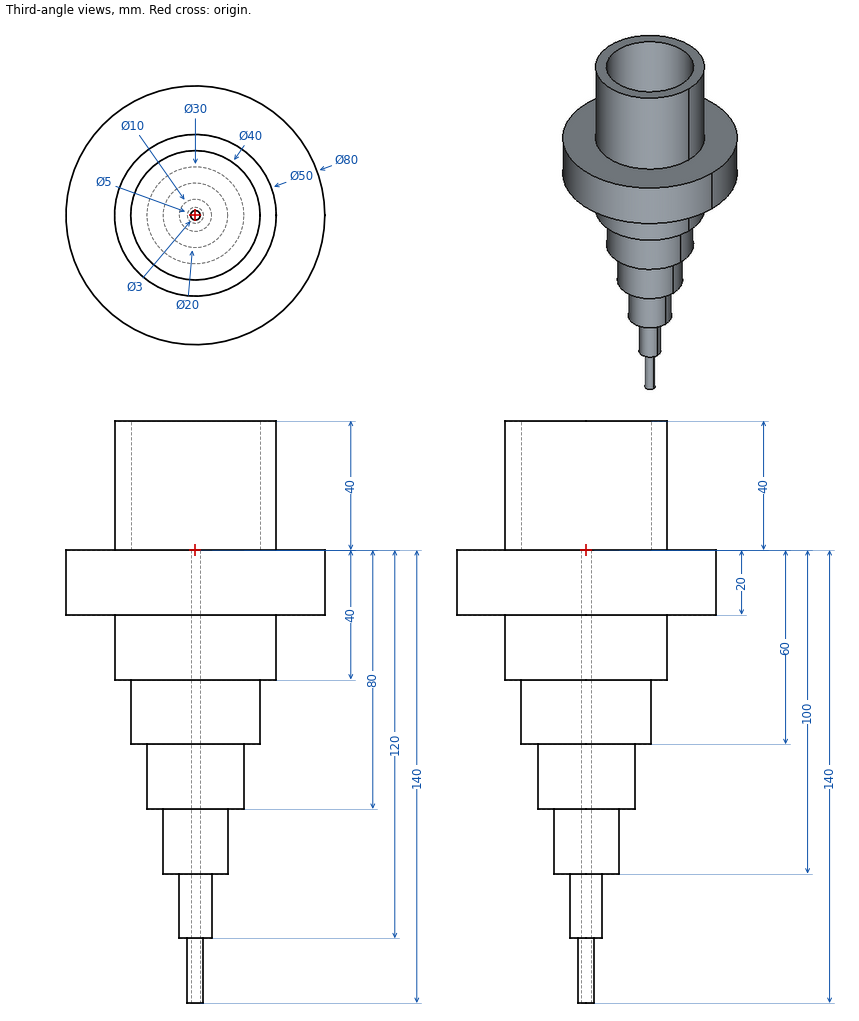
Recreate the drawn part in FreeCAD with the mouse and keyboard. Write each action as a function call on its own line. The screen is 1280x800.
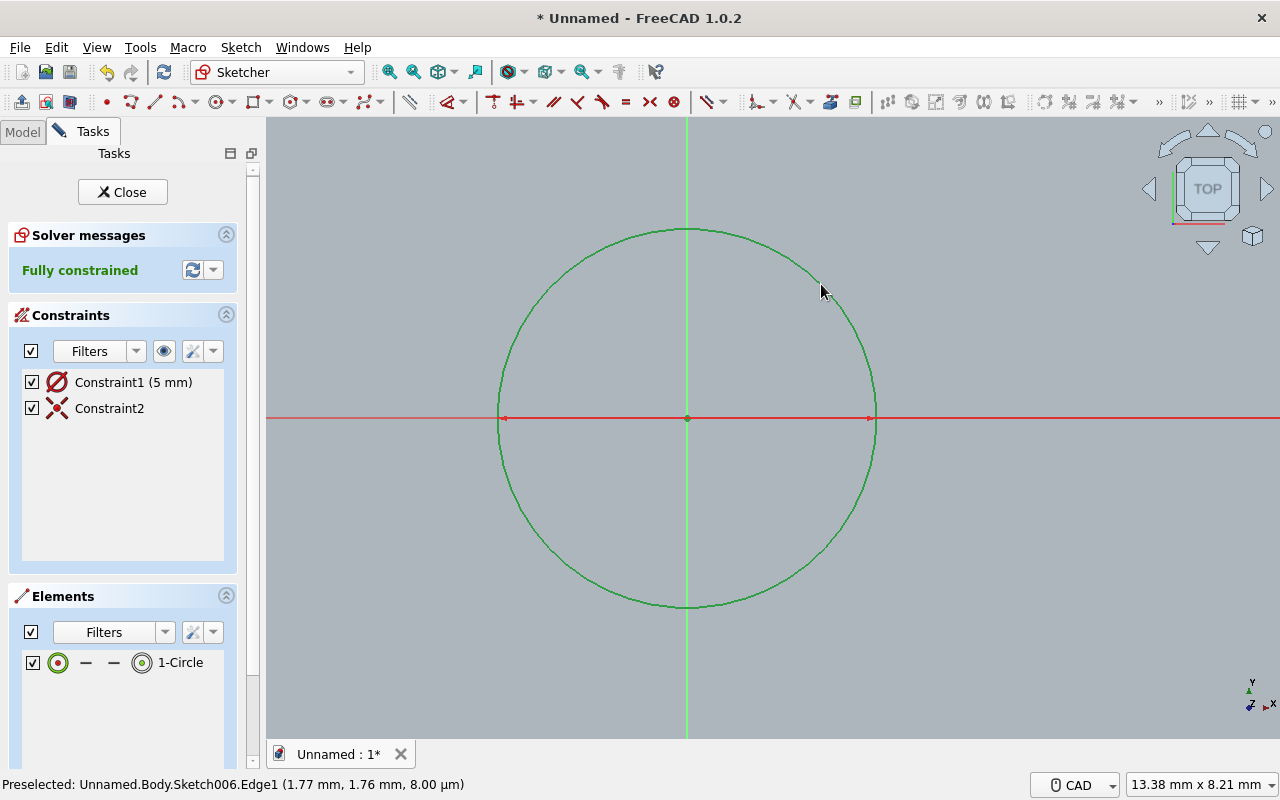
click(123, 192)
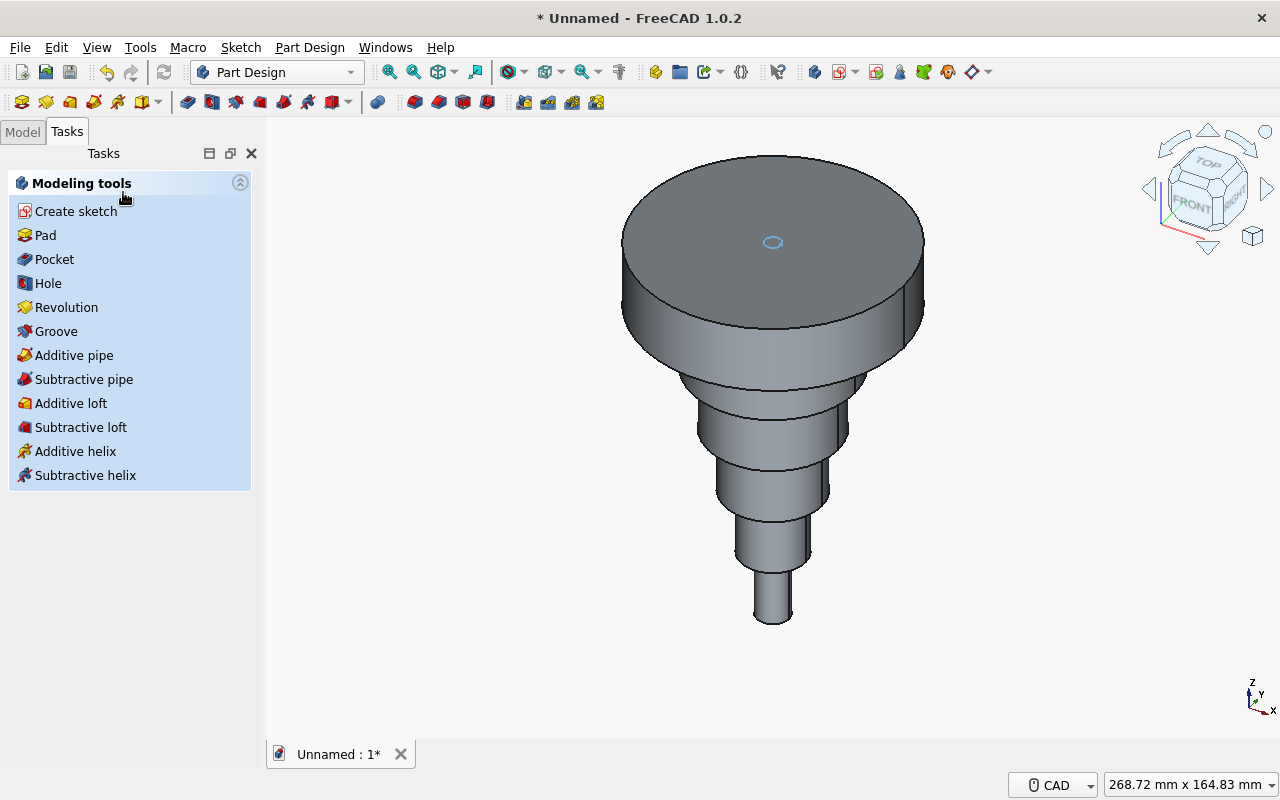
click(22, 102)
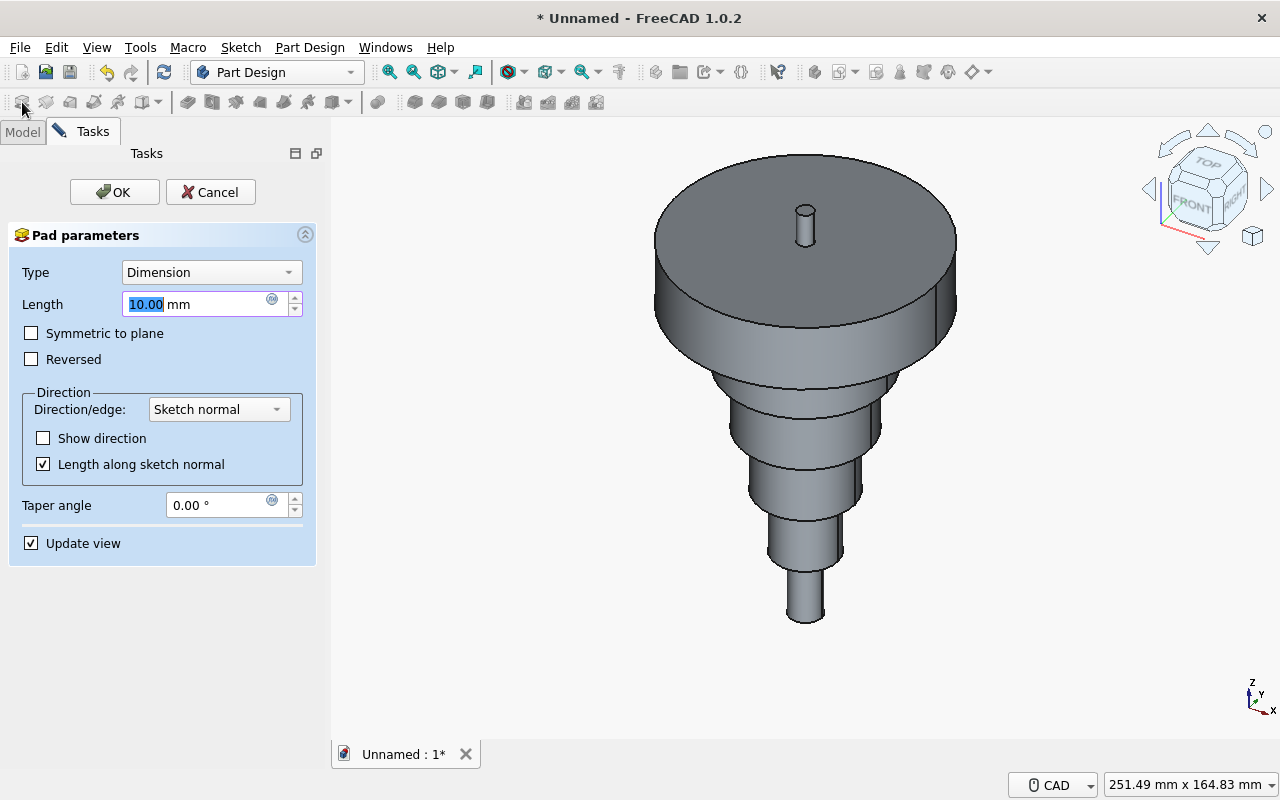
text(140)
key(Tab)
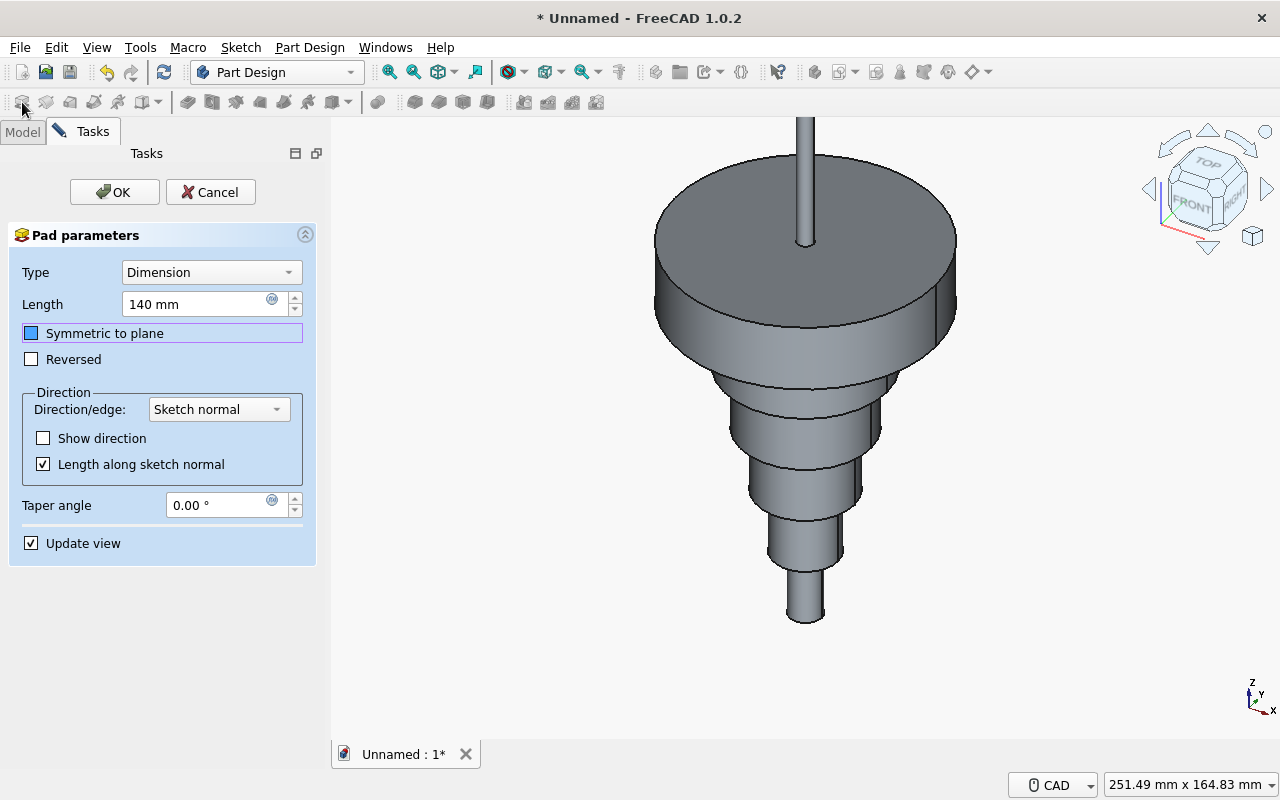
click(30, 359)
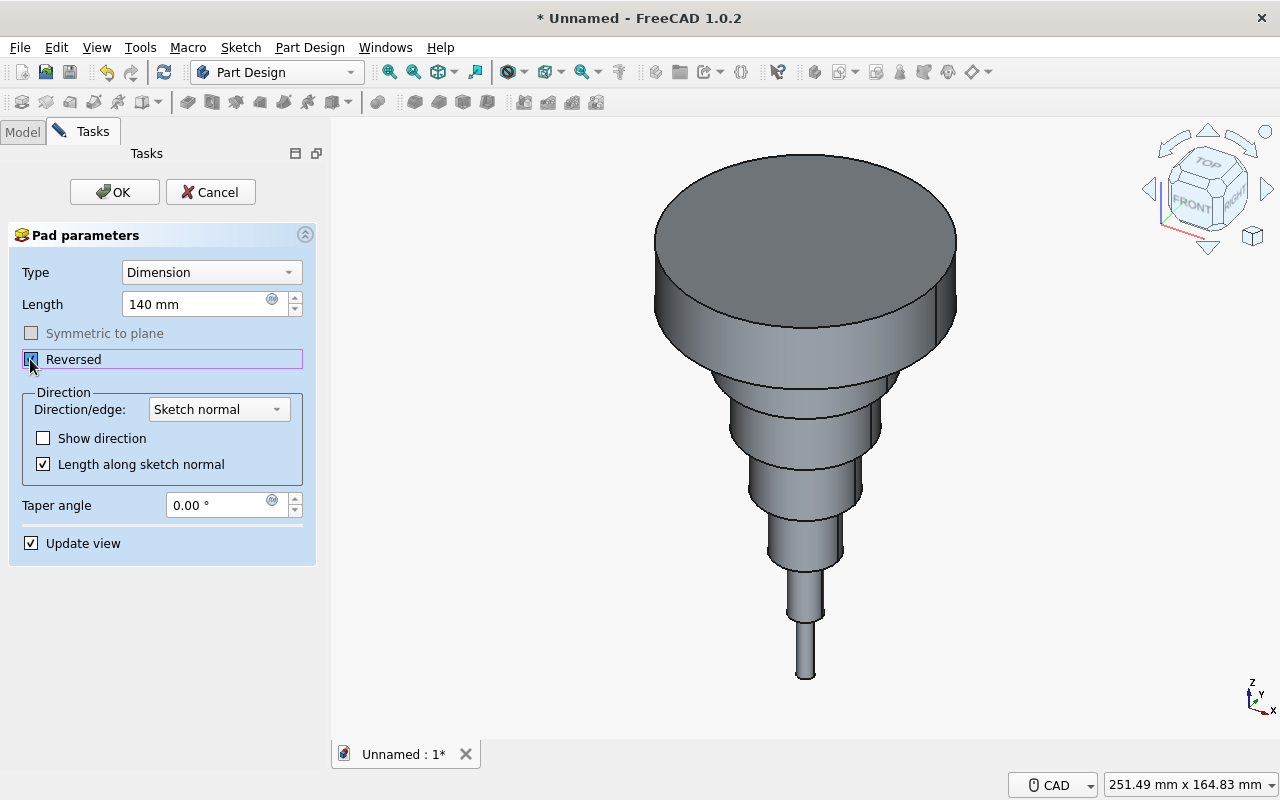
click(115, 192)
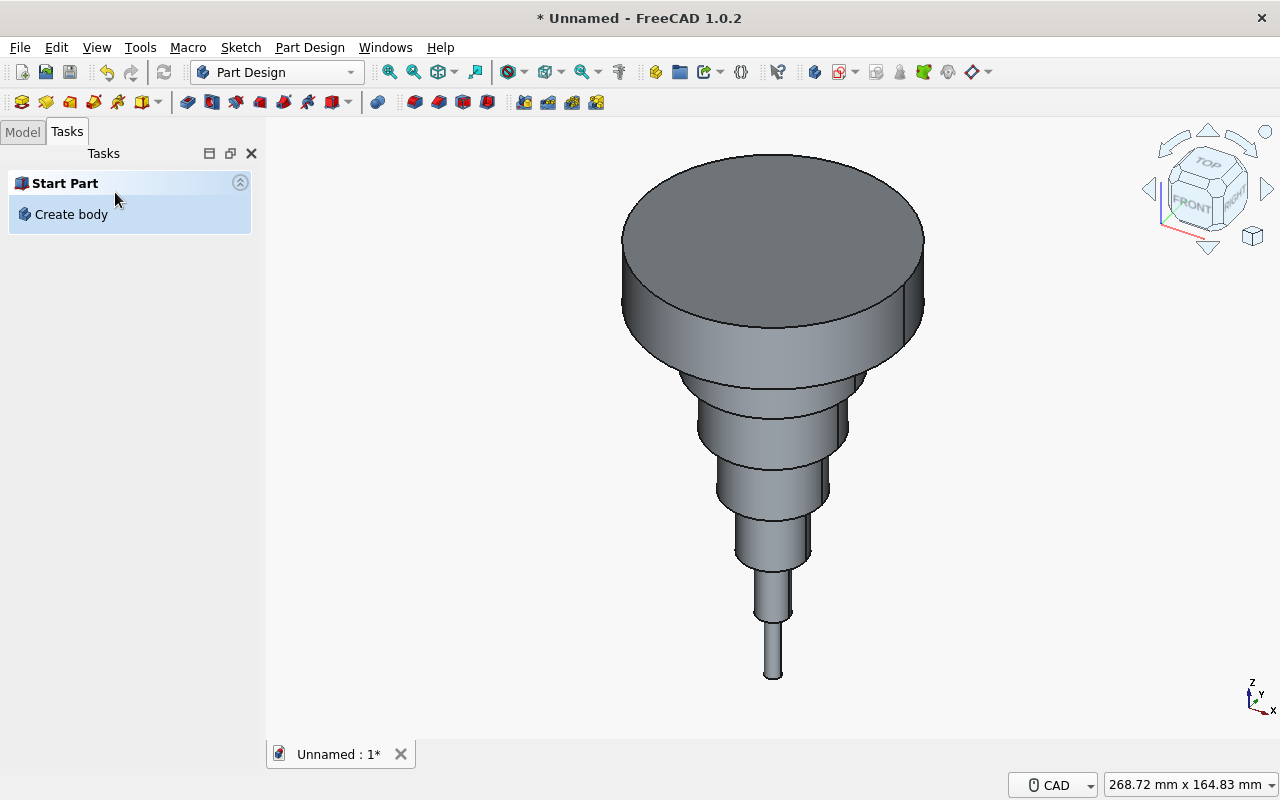
key(v)
key(f)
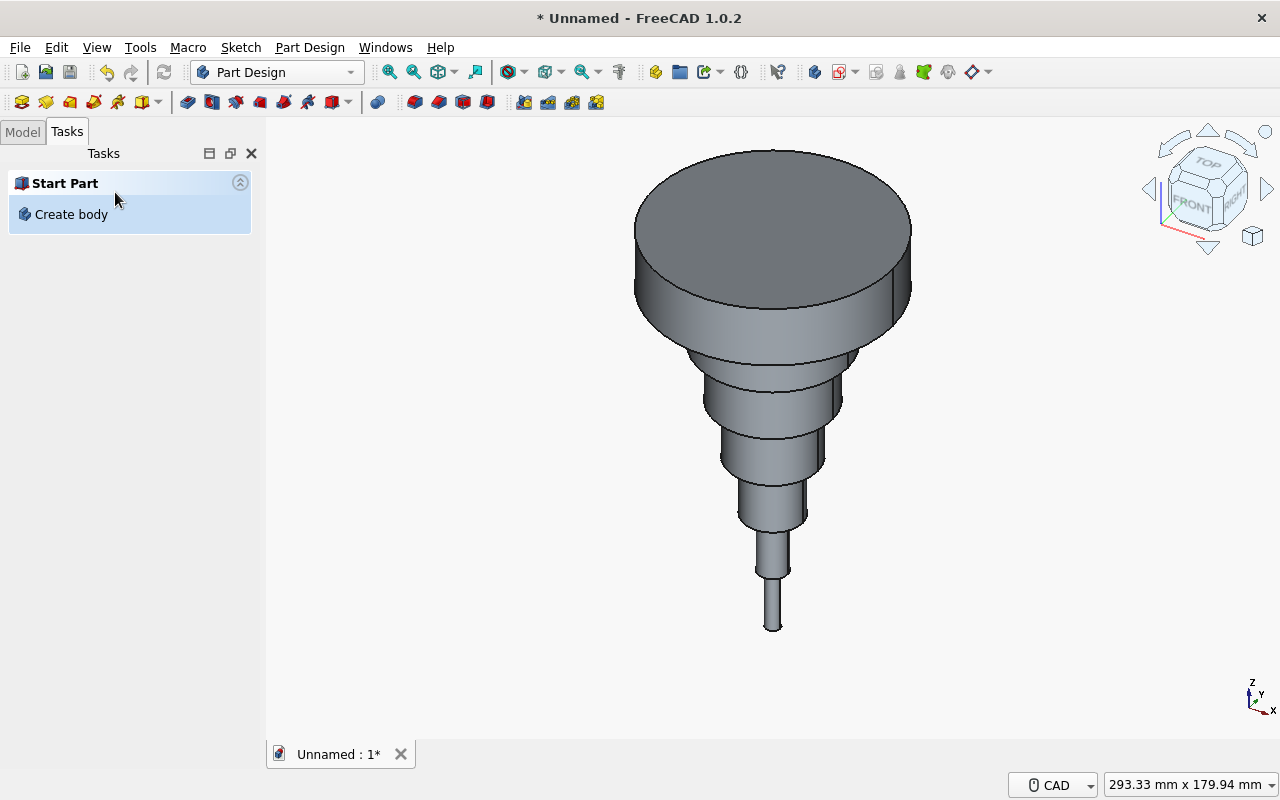
click(23, 131)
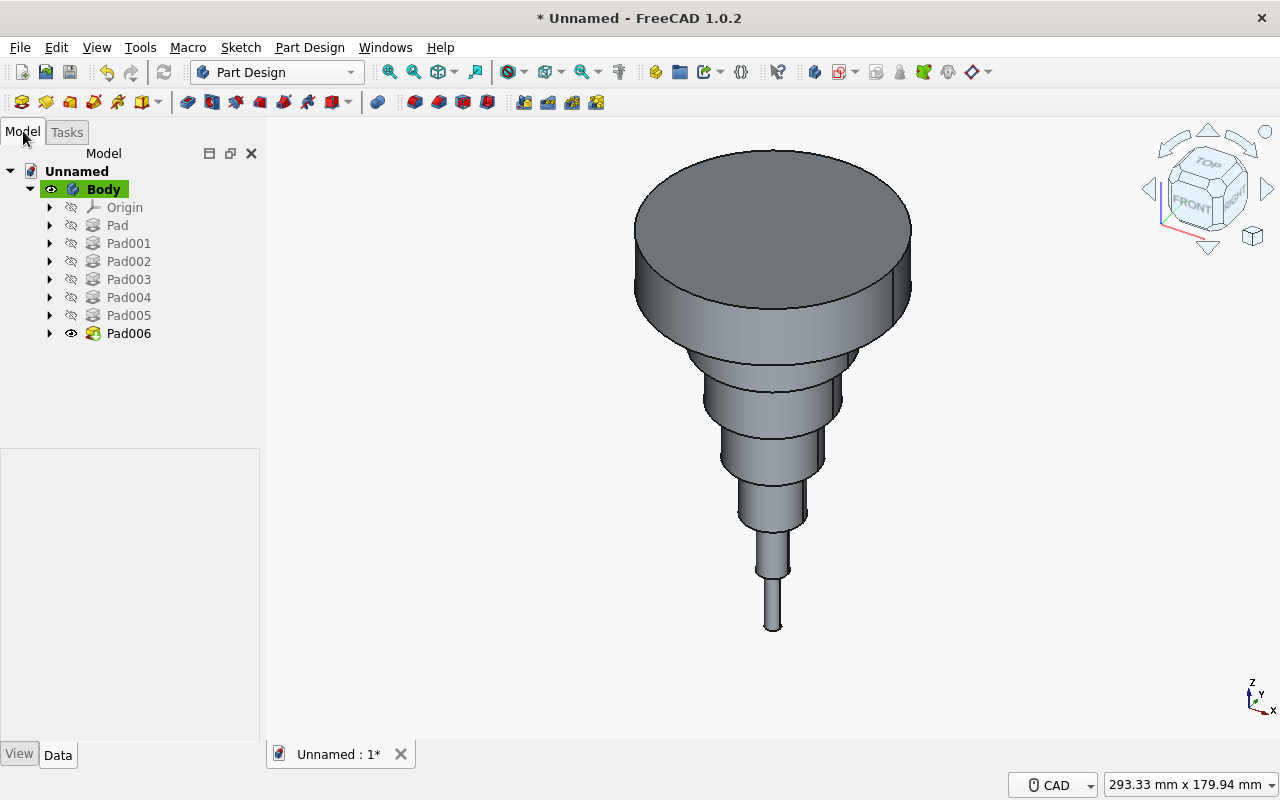
click(50, 207)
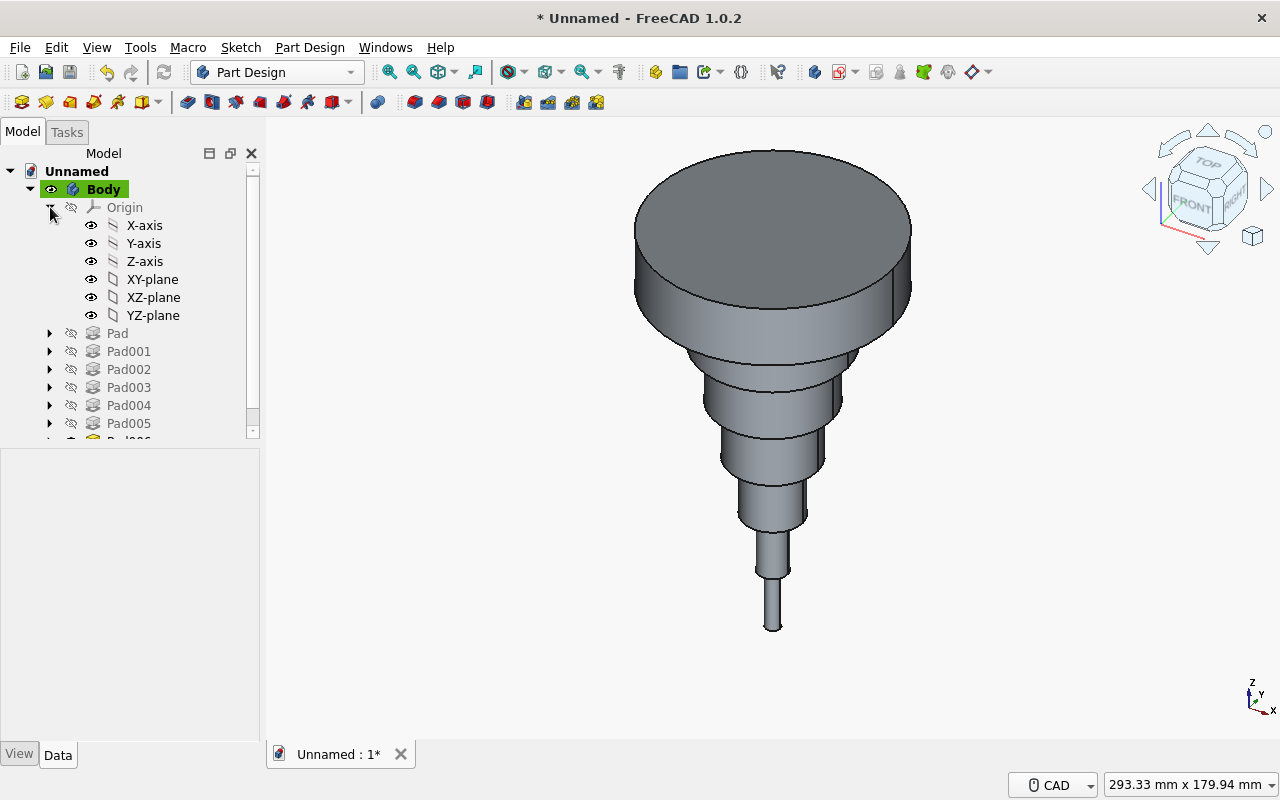
click(136, 279)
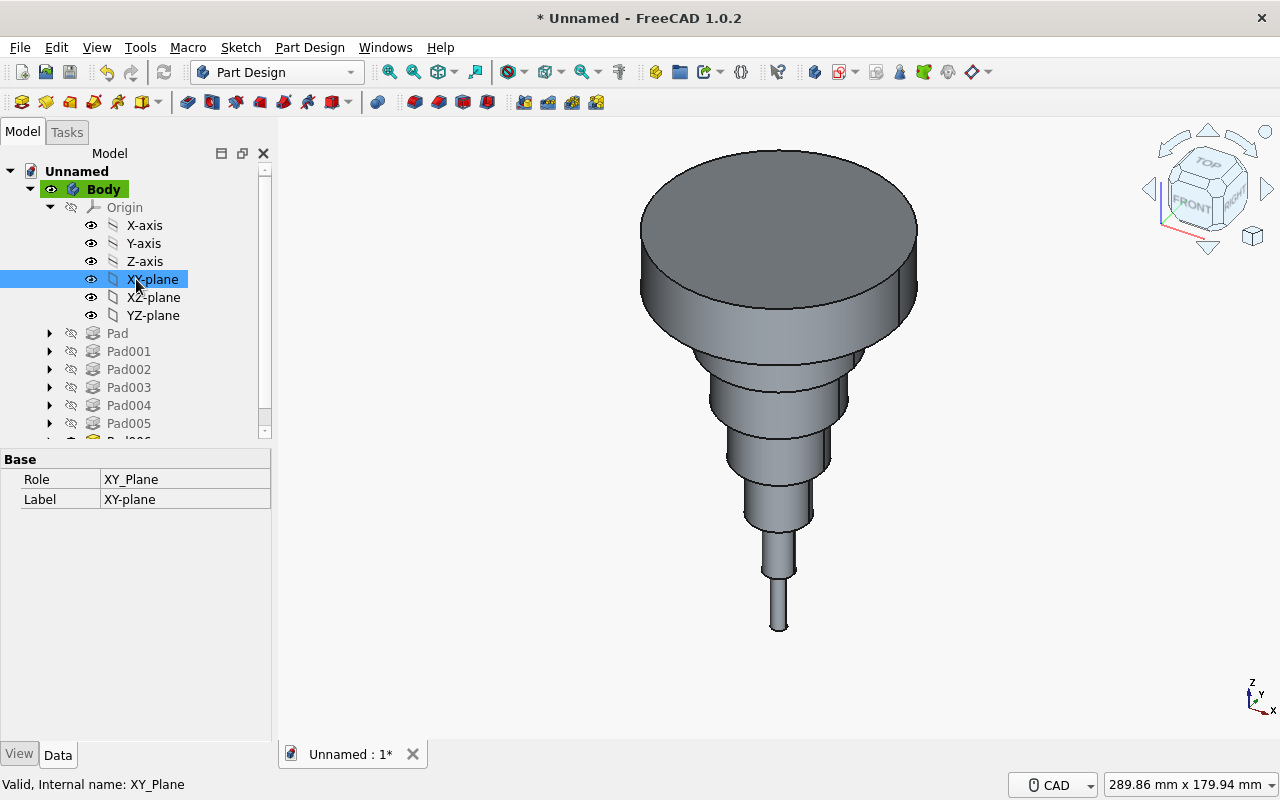
click(972, 72)